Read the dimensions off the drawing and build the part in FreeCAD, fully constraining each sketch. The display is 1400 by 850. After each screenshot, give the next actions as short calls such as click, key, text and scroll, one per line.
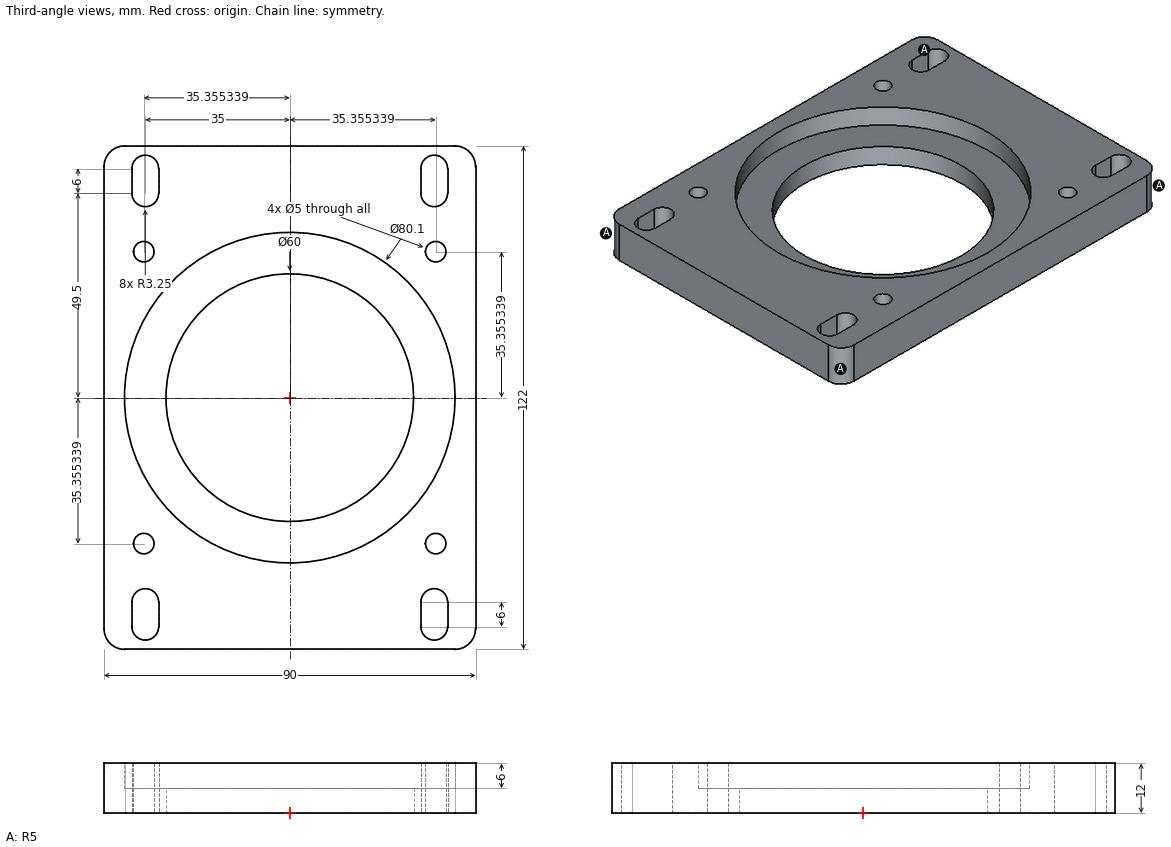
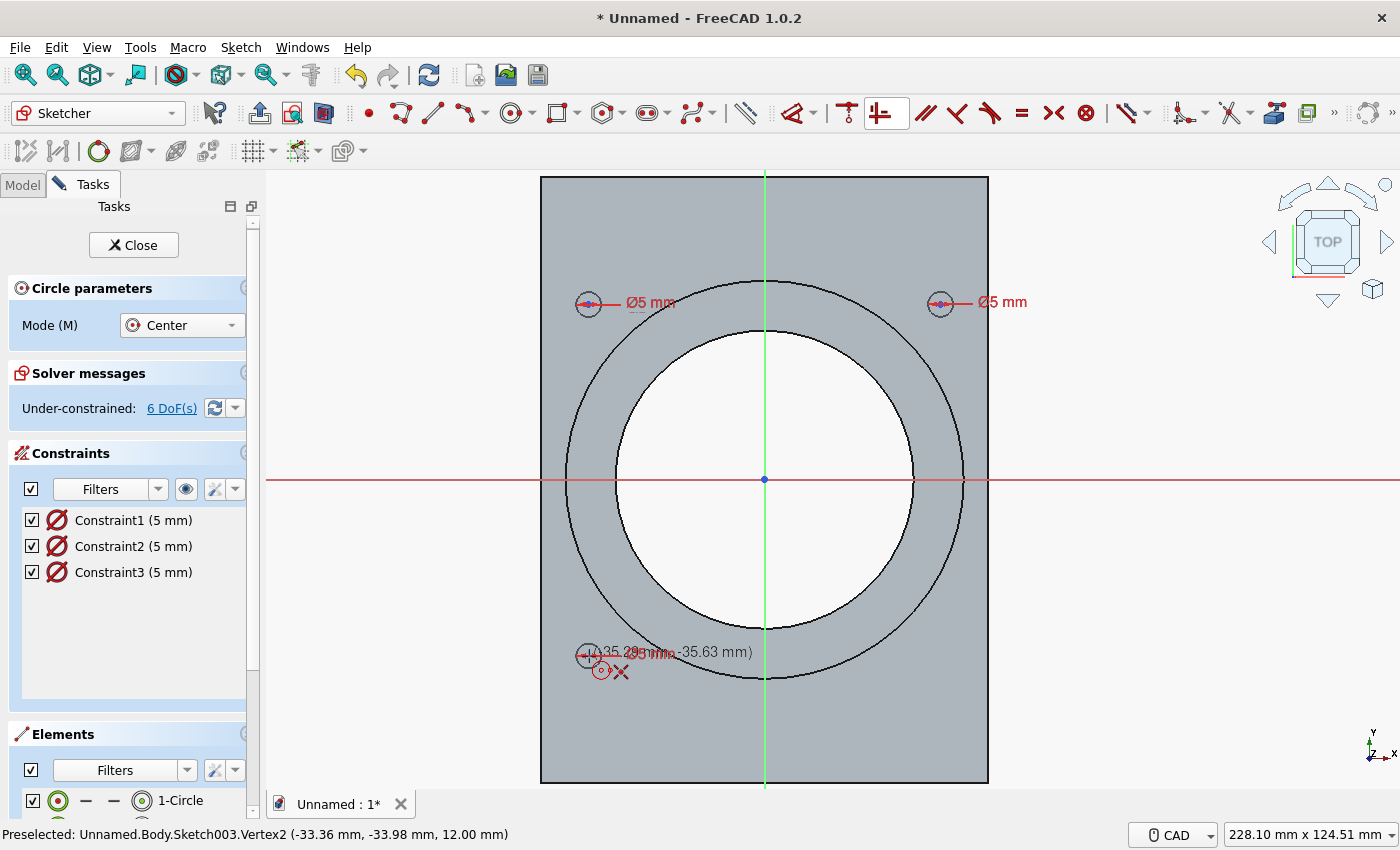
scroll(940, 656, up, 4)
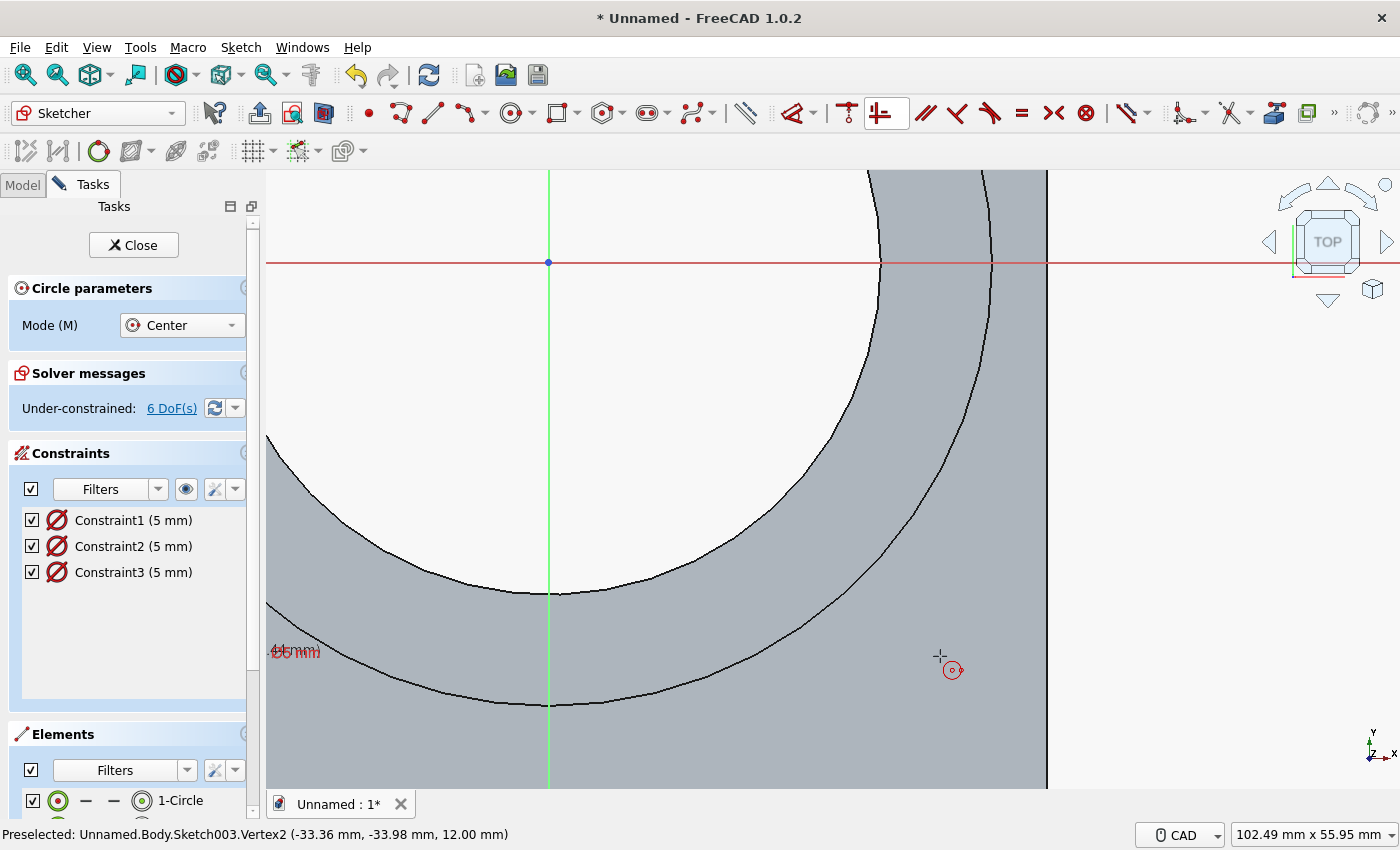
click(940, 654)
move(960, 634)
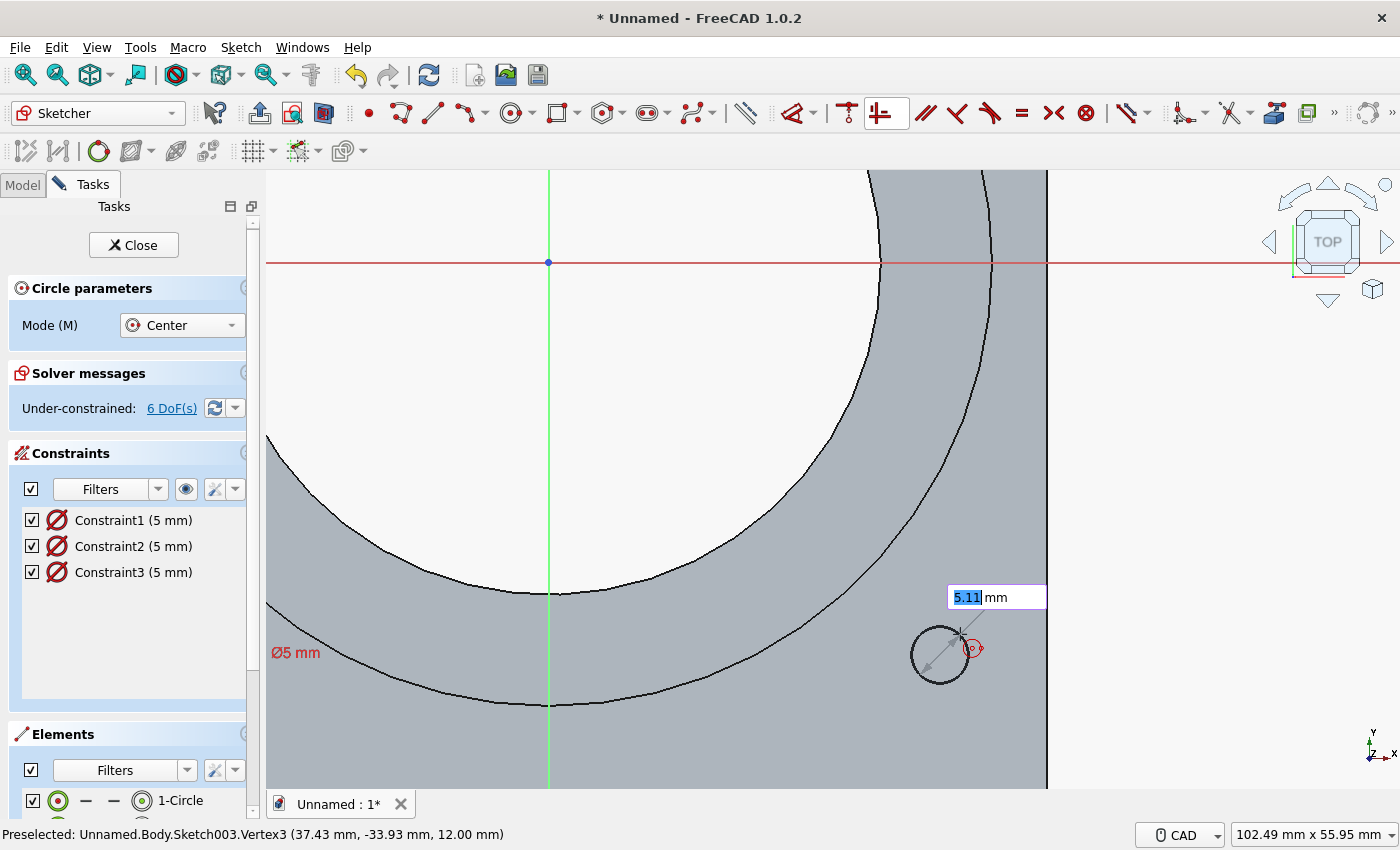
text(5)
key(Return)
key(Escape)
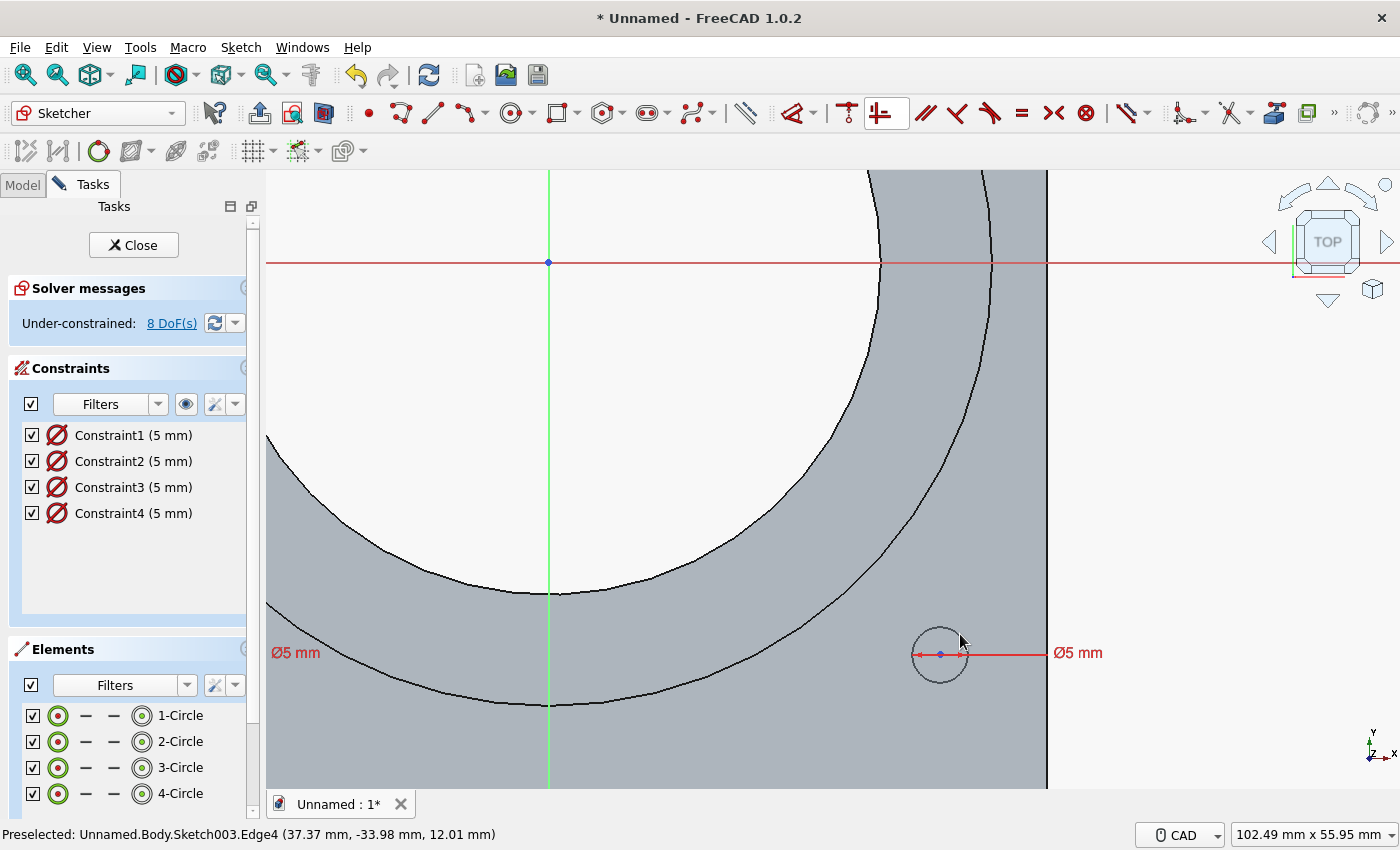
scroll(940, 656, down, 4)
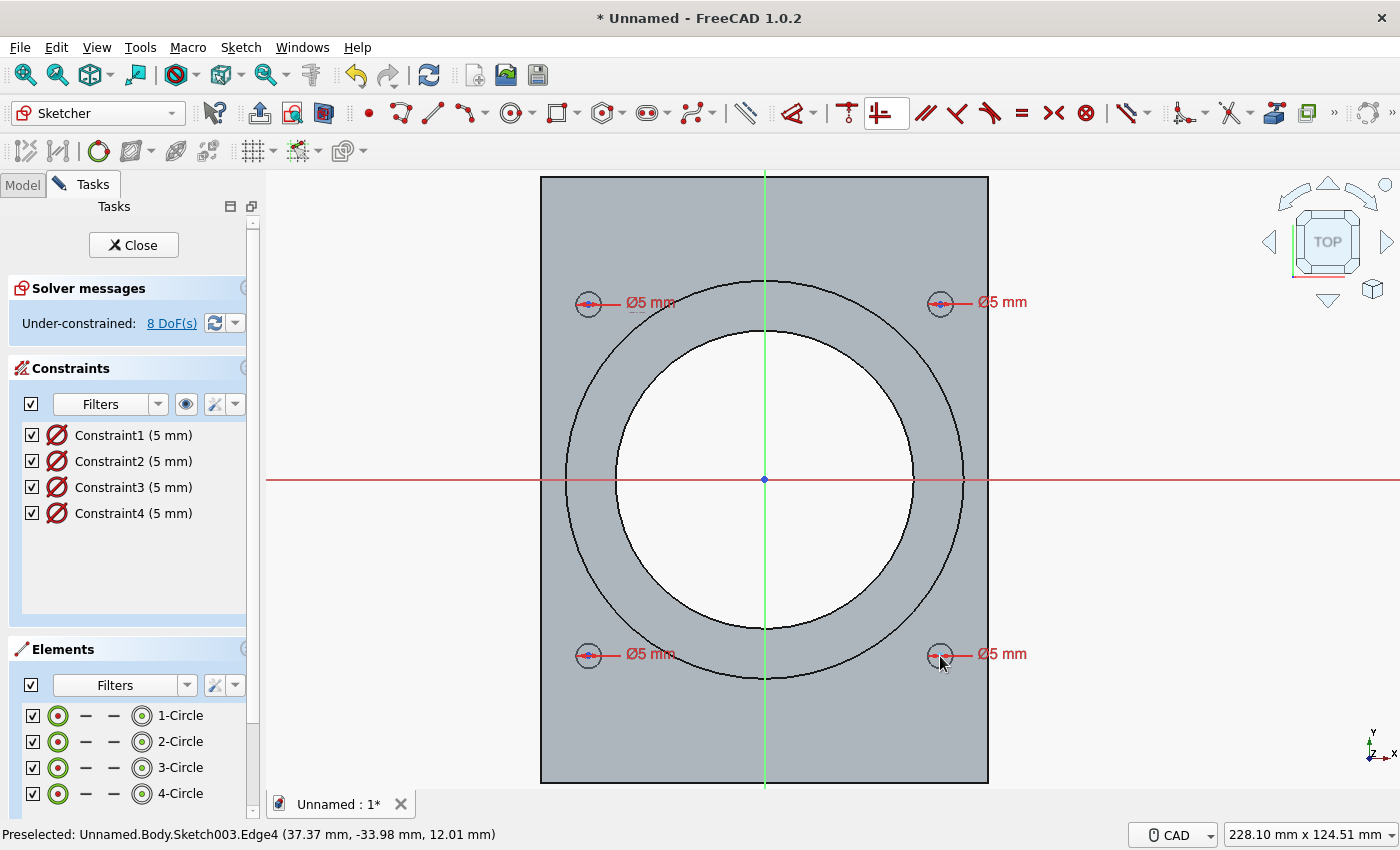
click(941, 304)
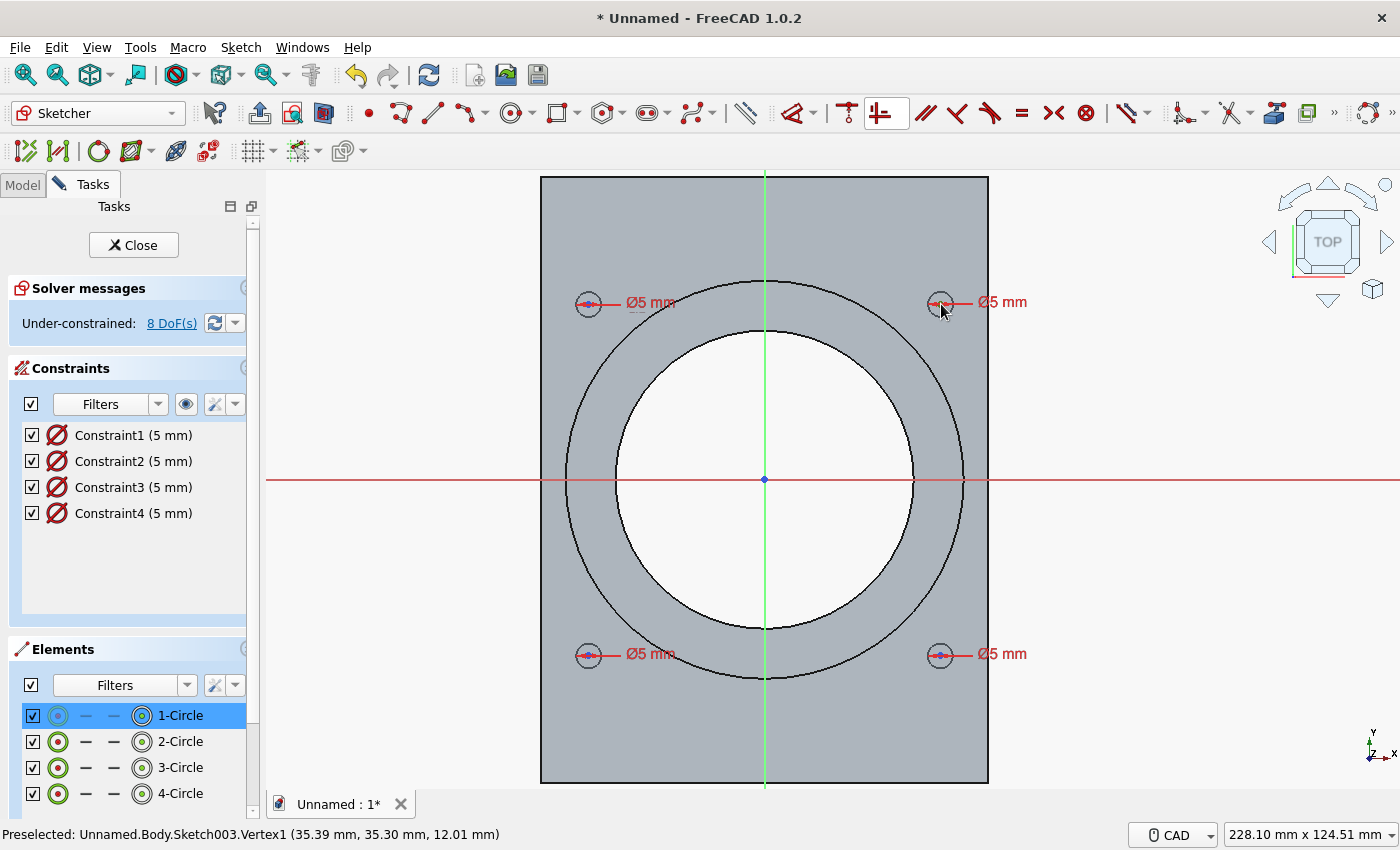
click(589, 305)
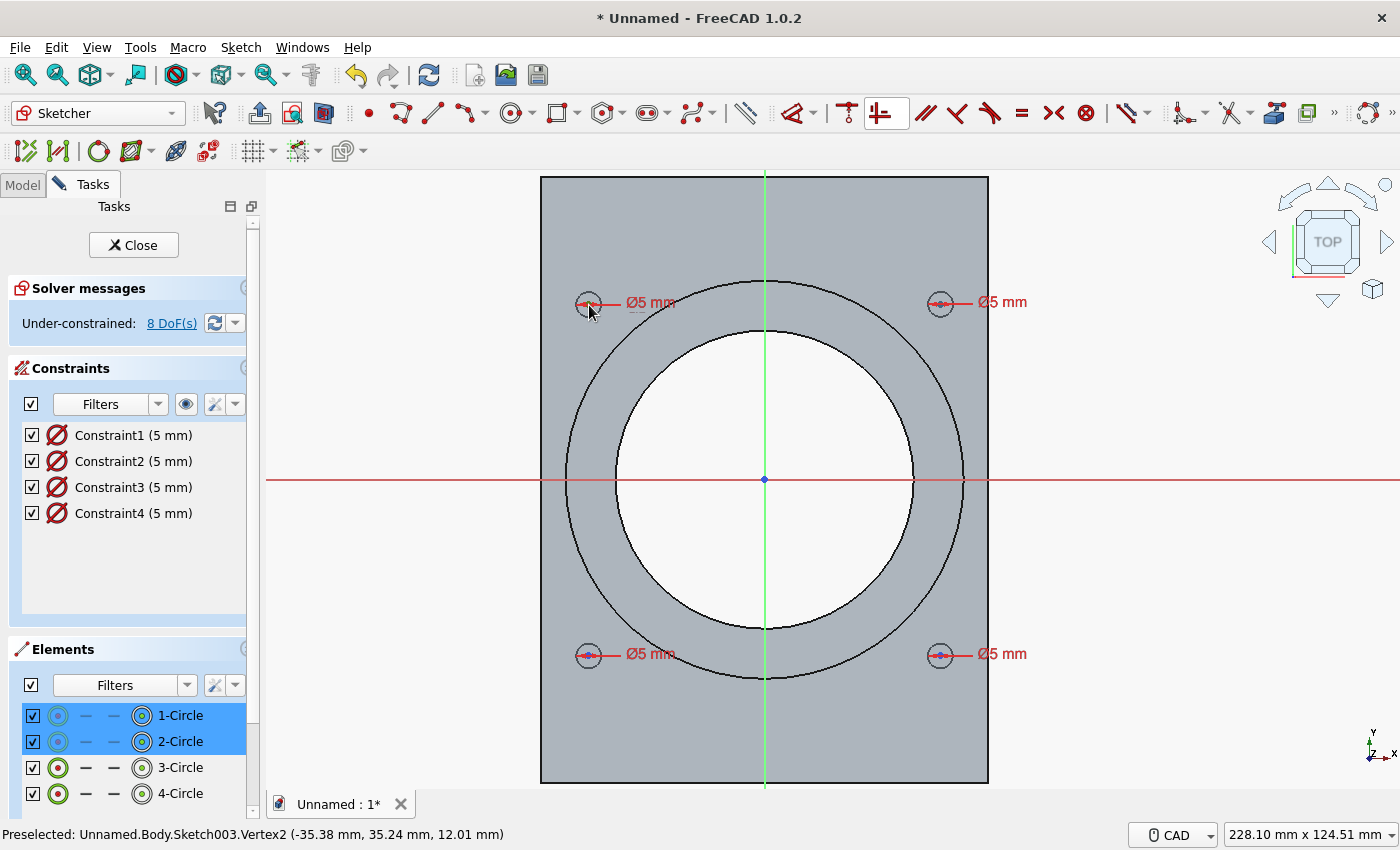
key(h)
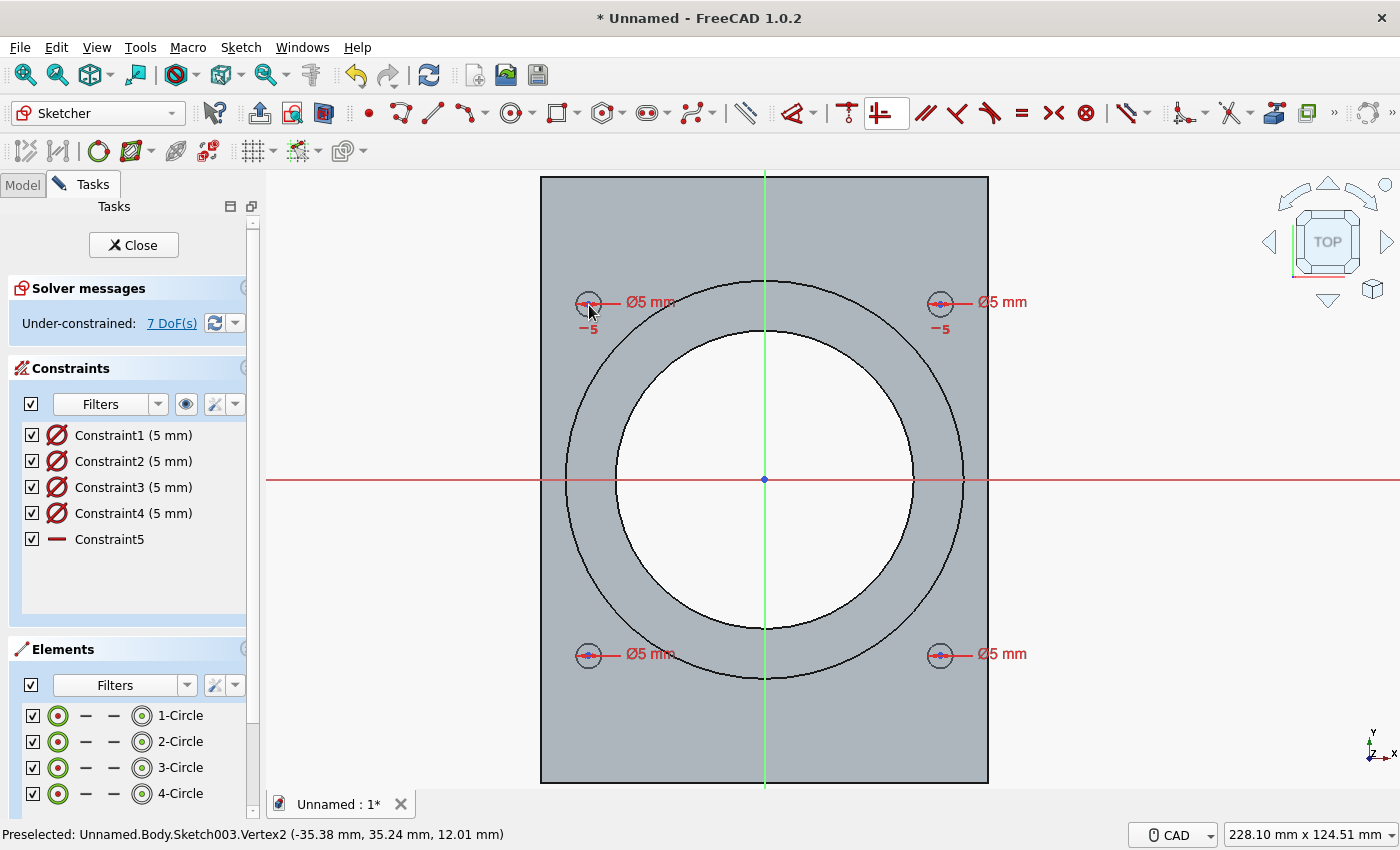
click(589, 304)